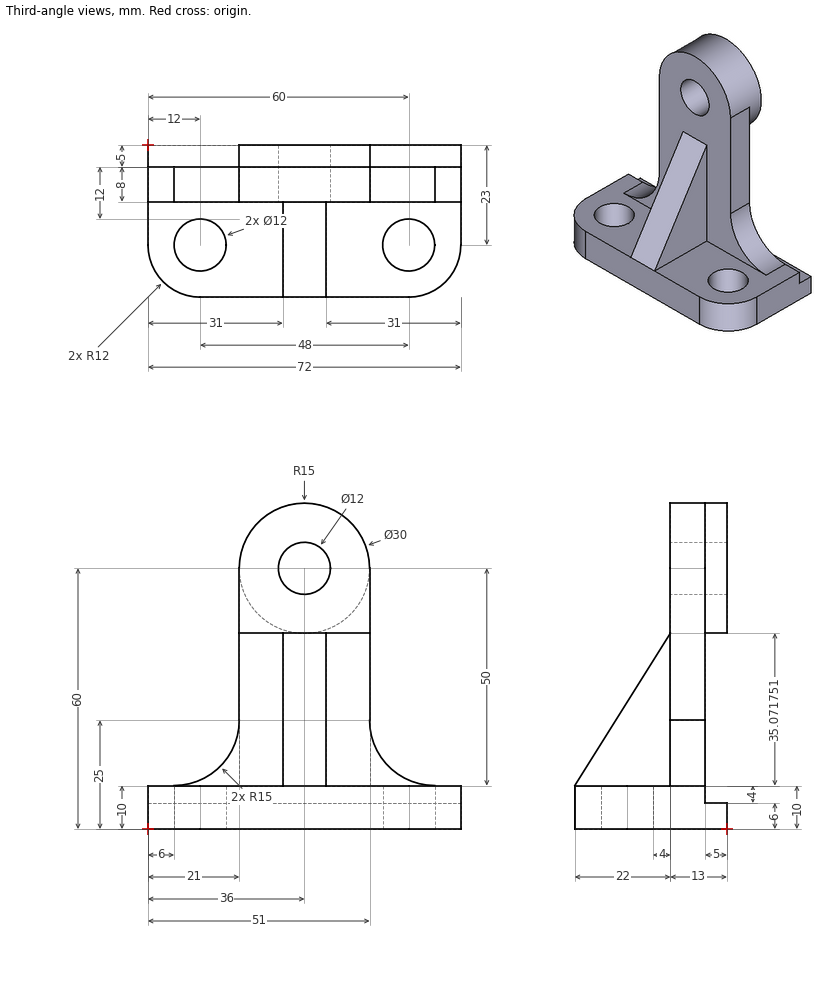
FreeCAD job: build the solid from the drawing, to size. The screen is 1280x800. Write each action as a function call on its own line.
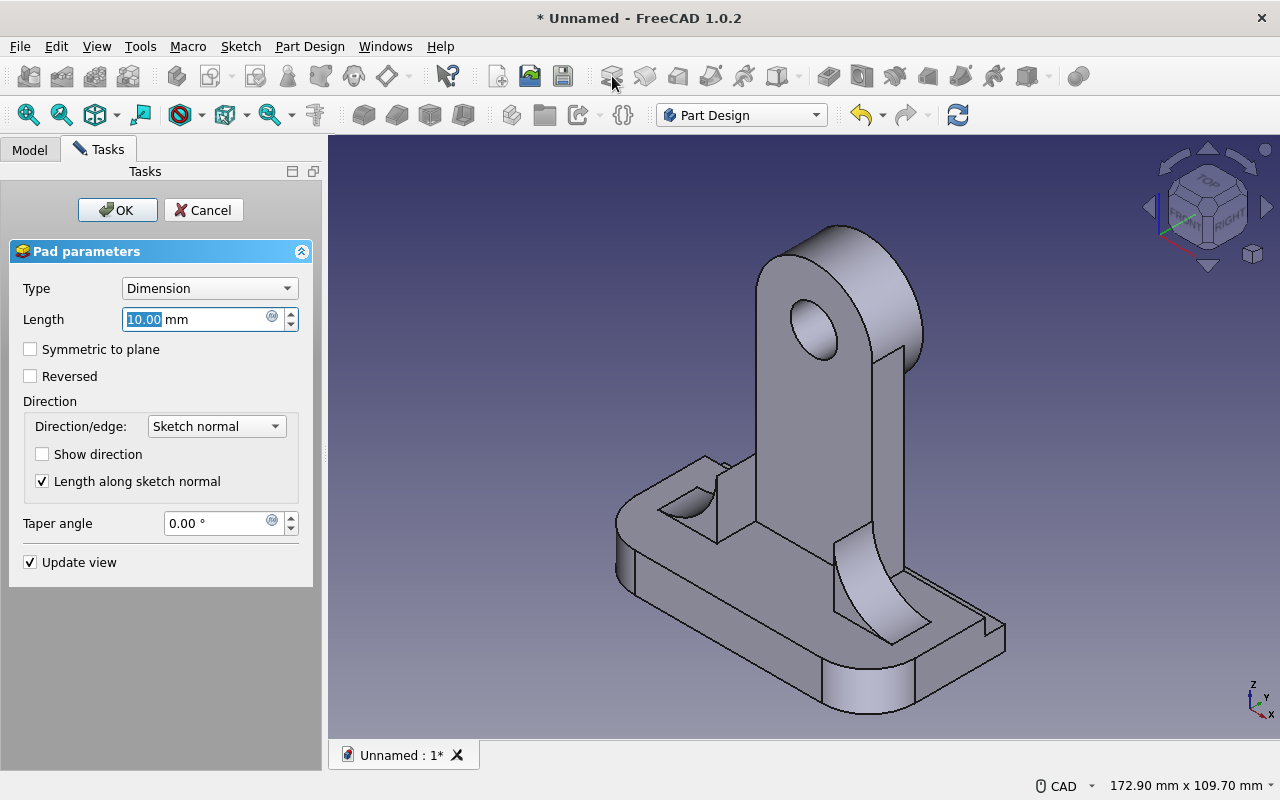
text(8)
key(Tab)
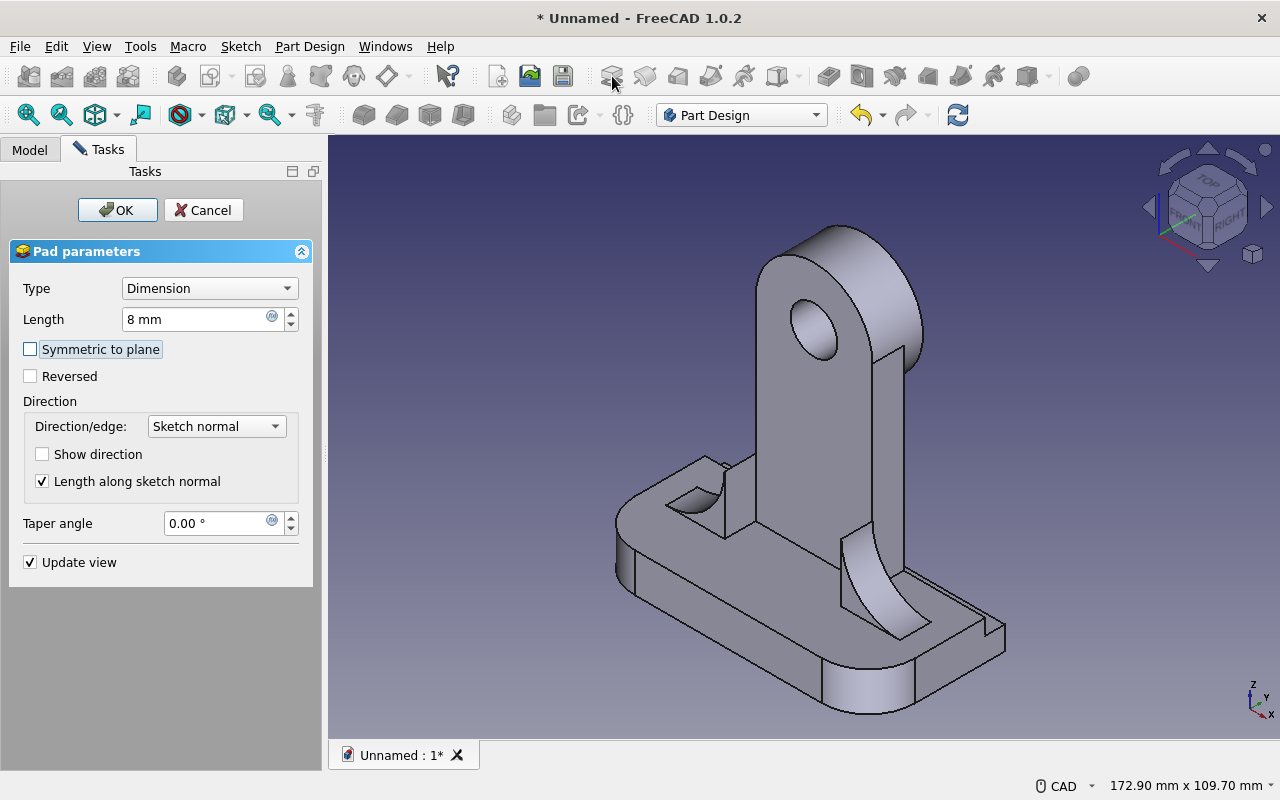
click(31, 376)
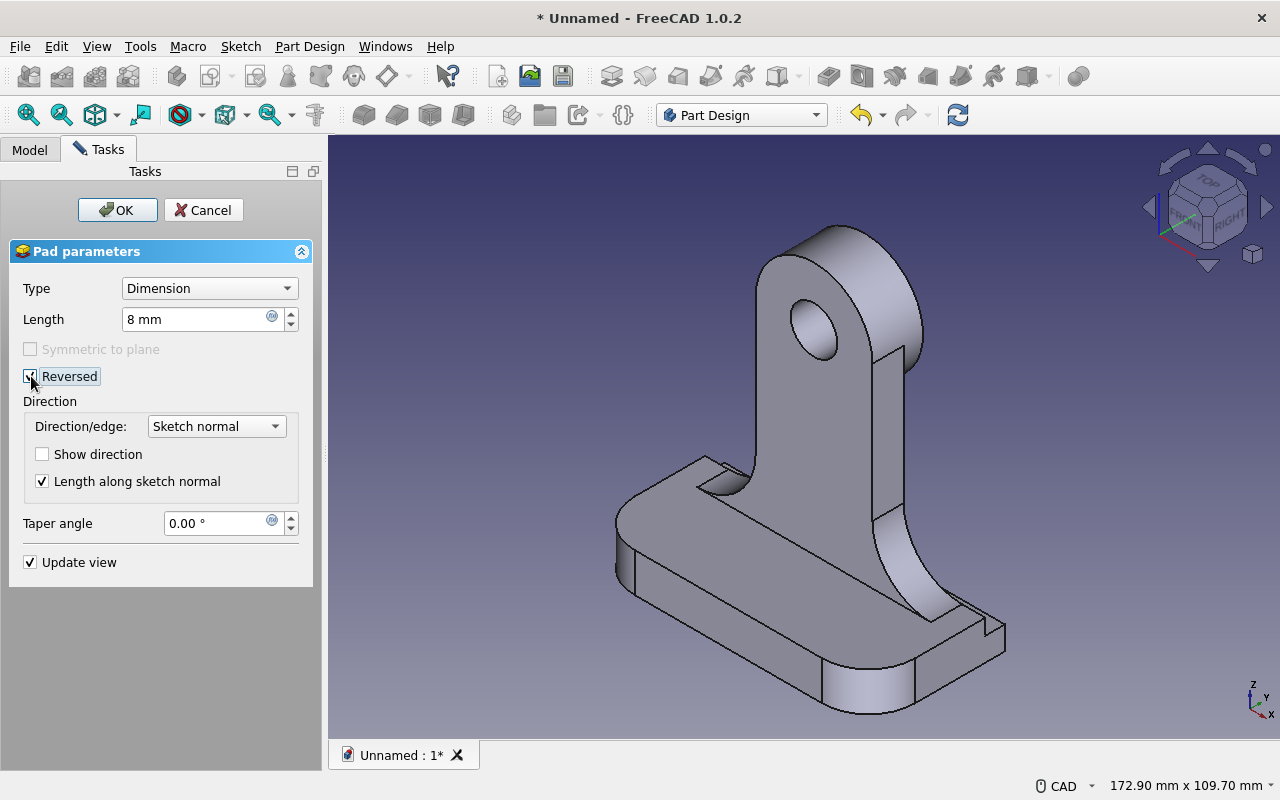
click(118, 210)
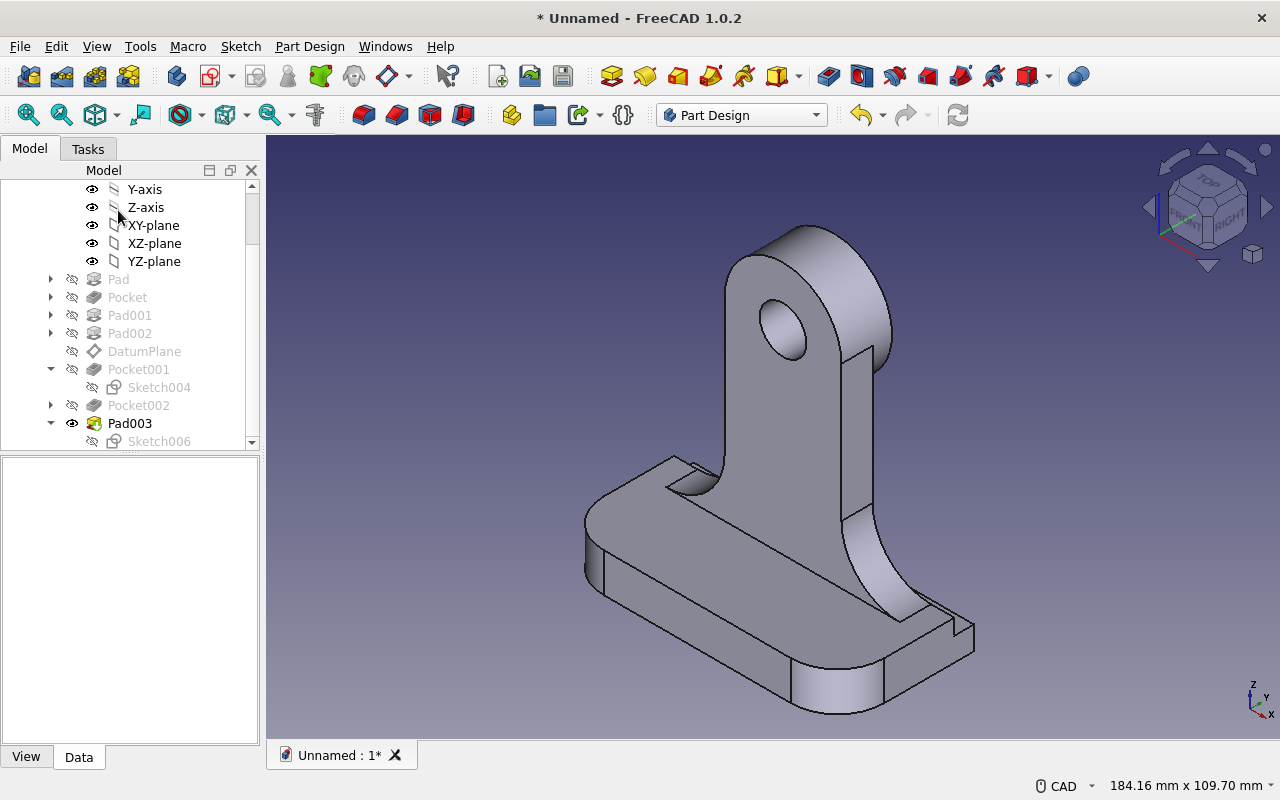
click(819, 625)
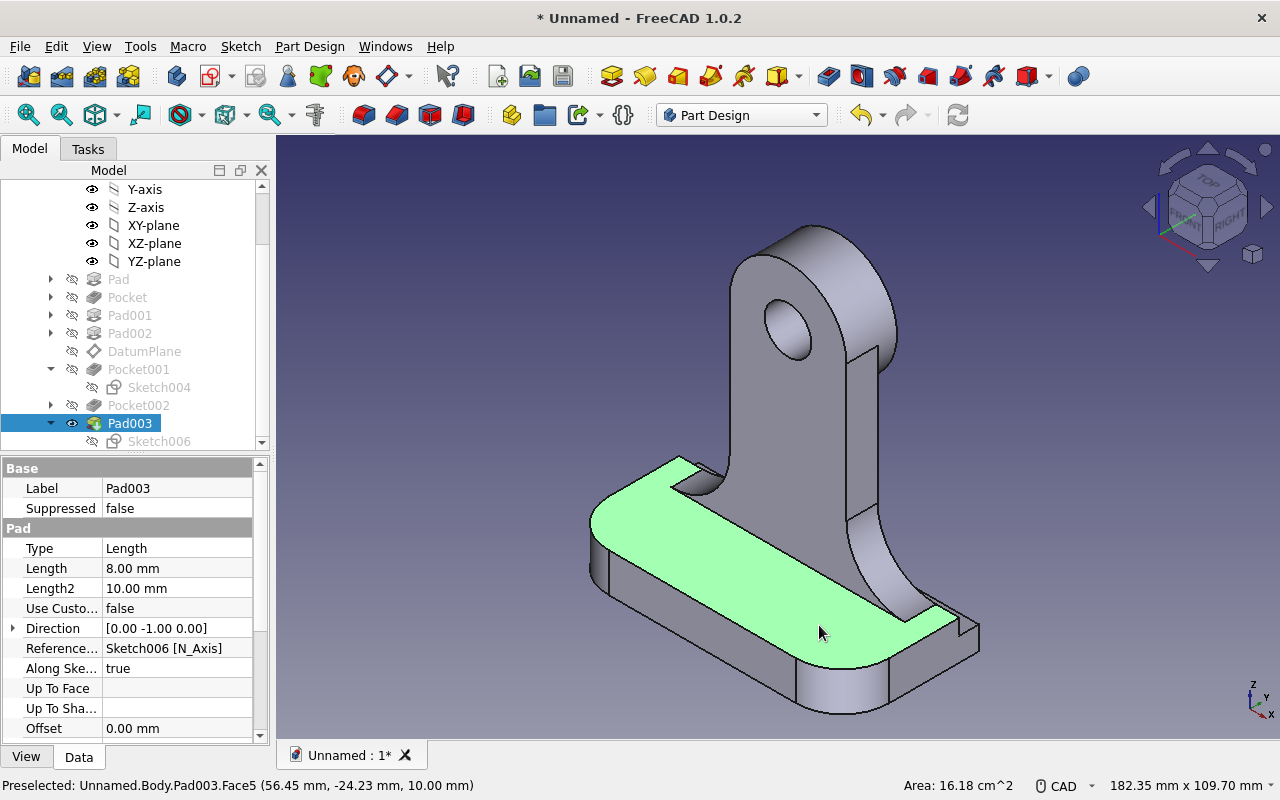
click(210, 76)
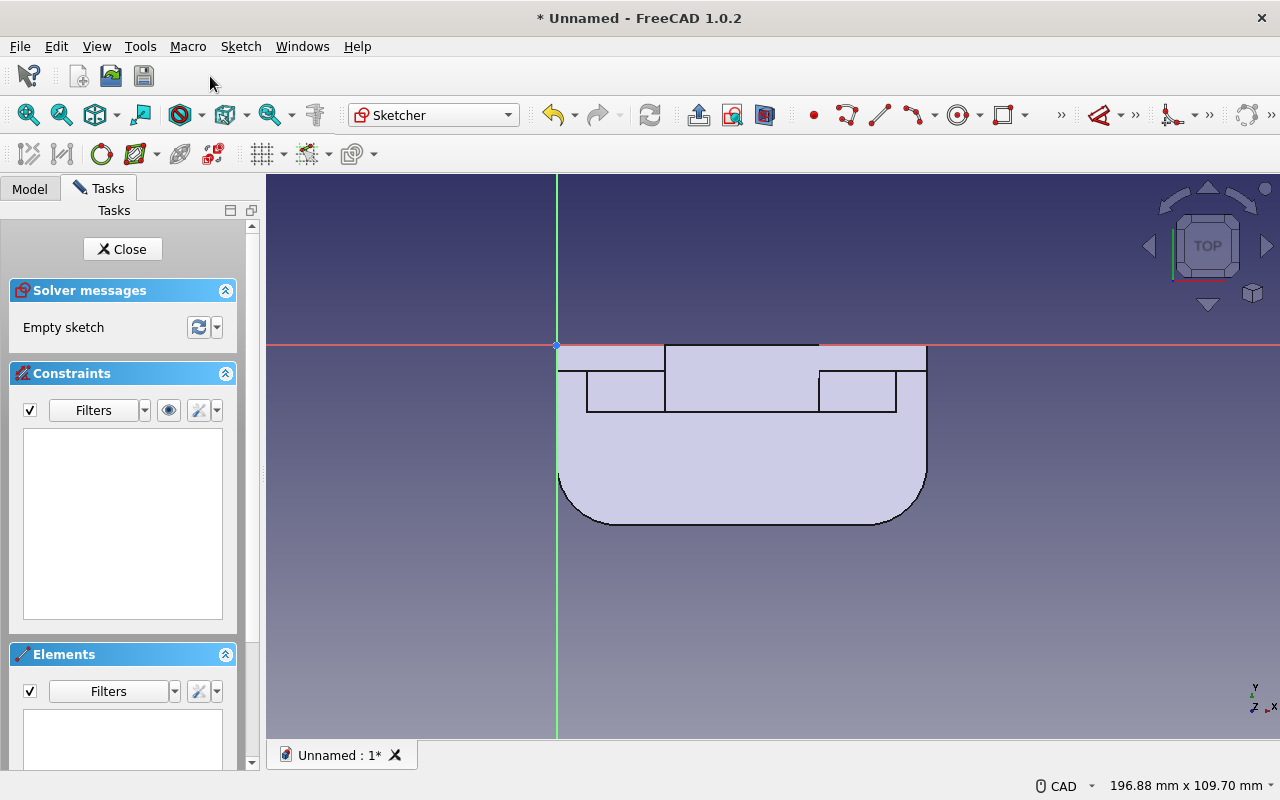
key(q)
key(s)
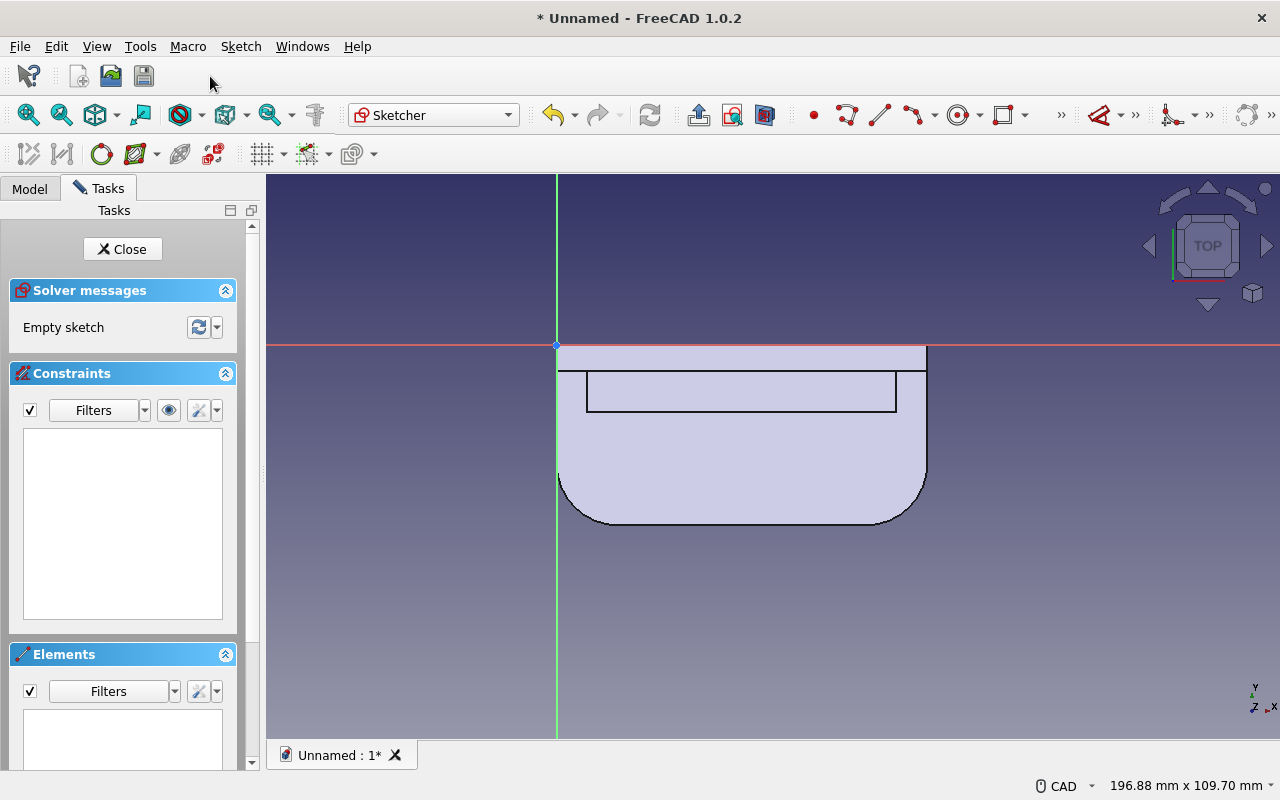
scroll(753, 375, up, 3)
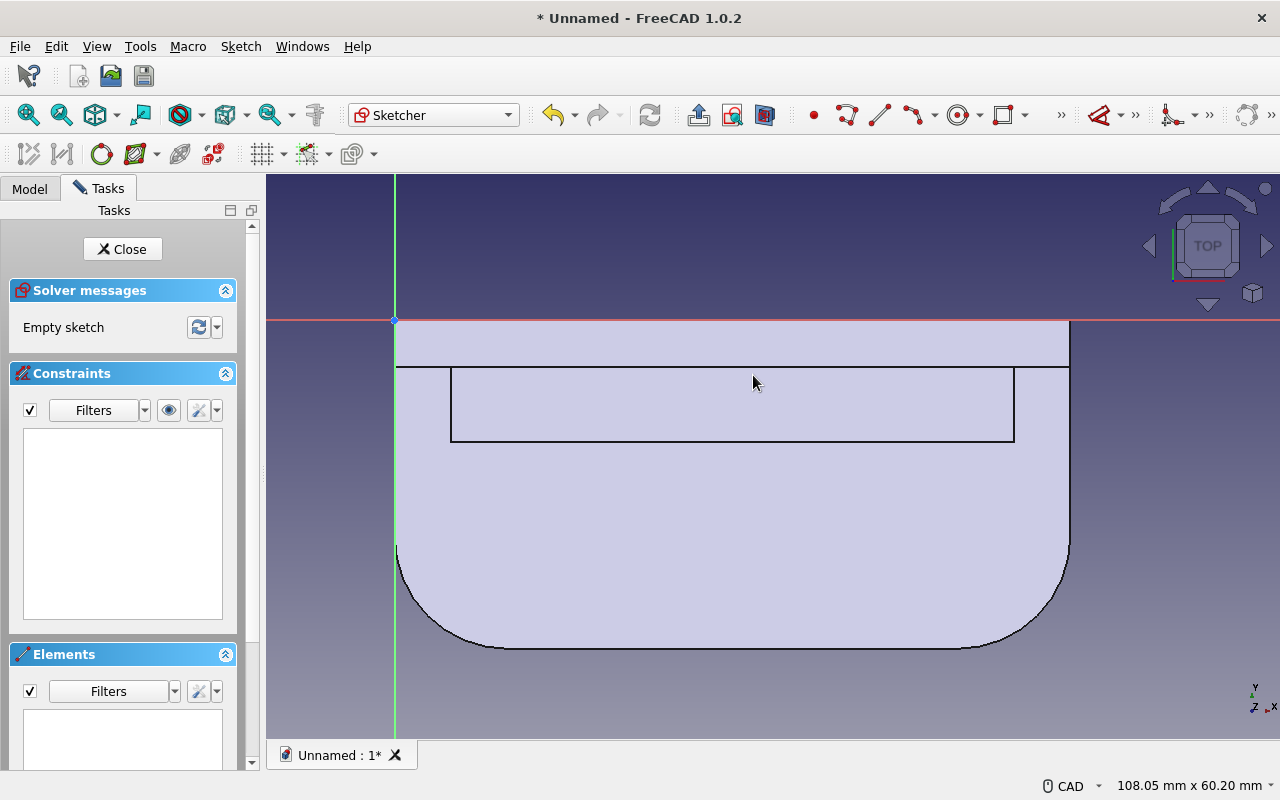
click(958, 116)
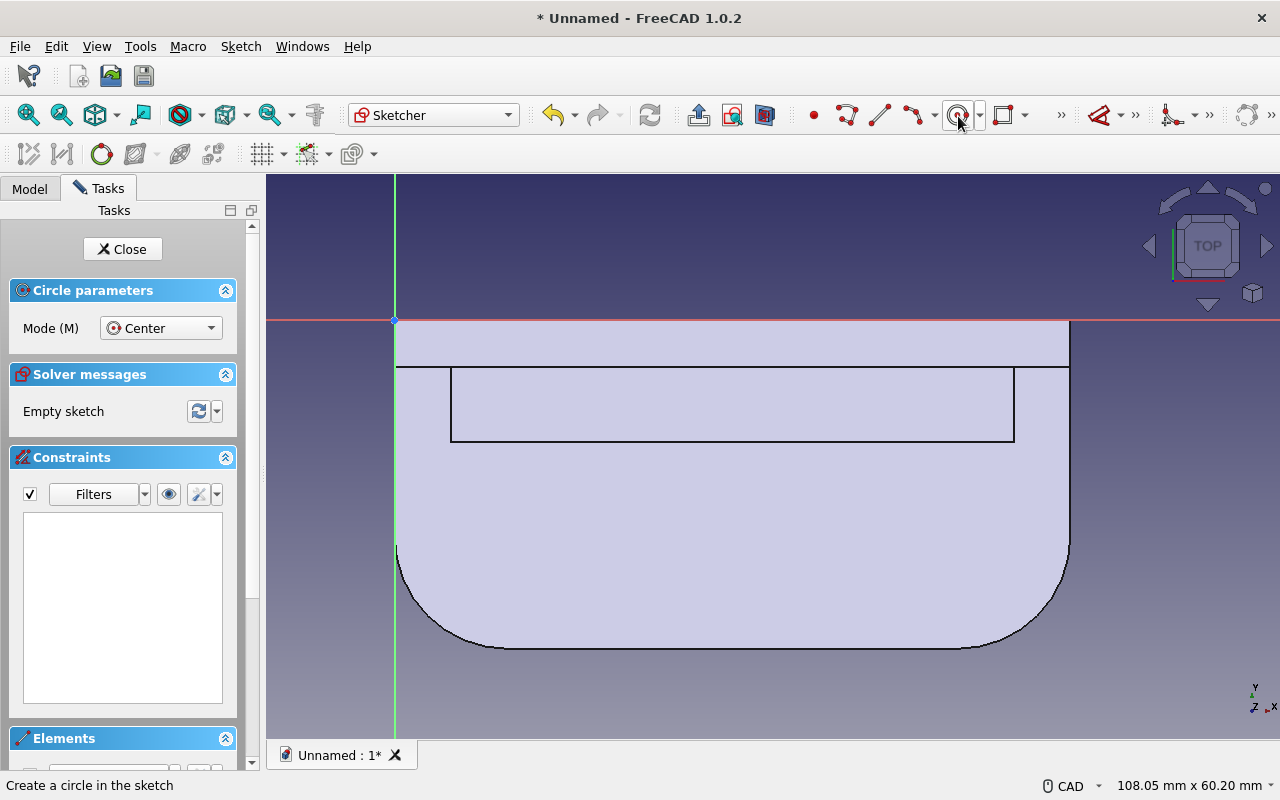
click(507, 536)
click(547, 496)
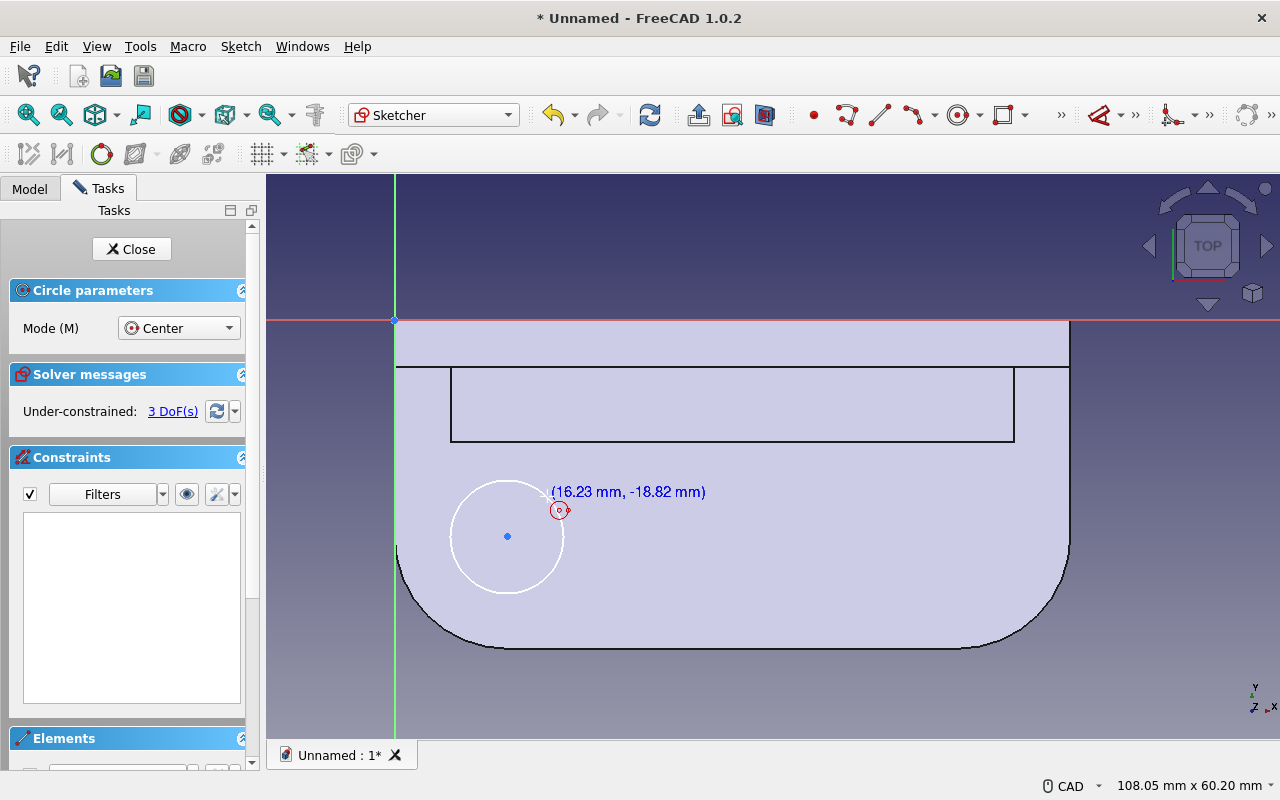
click(958, 536)
click(998, 496)
key(Escape)